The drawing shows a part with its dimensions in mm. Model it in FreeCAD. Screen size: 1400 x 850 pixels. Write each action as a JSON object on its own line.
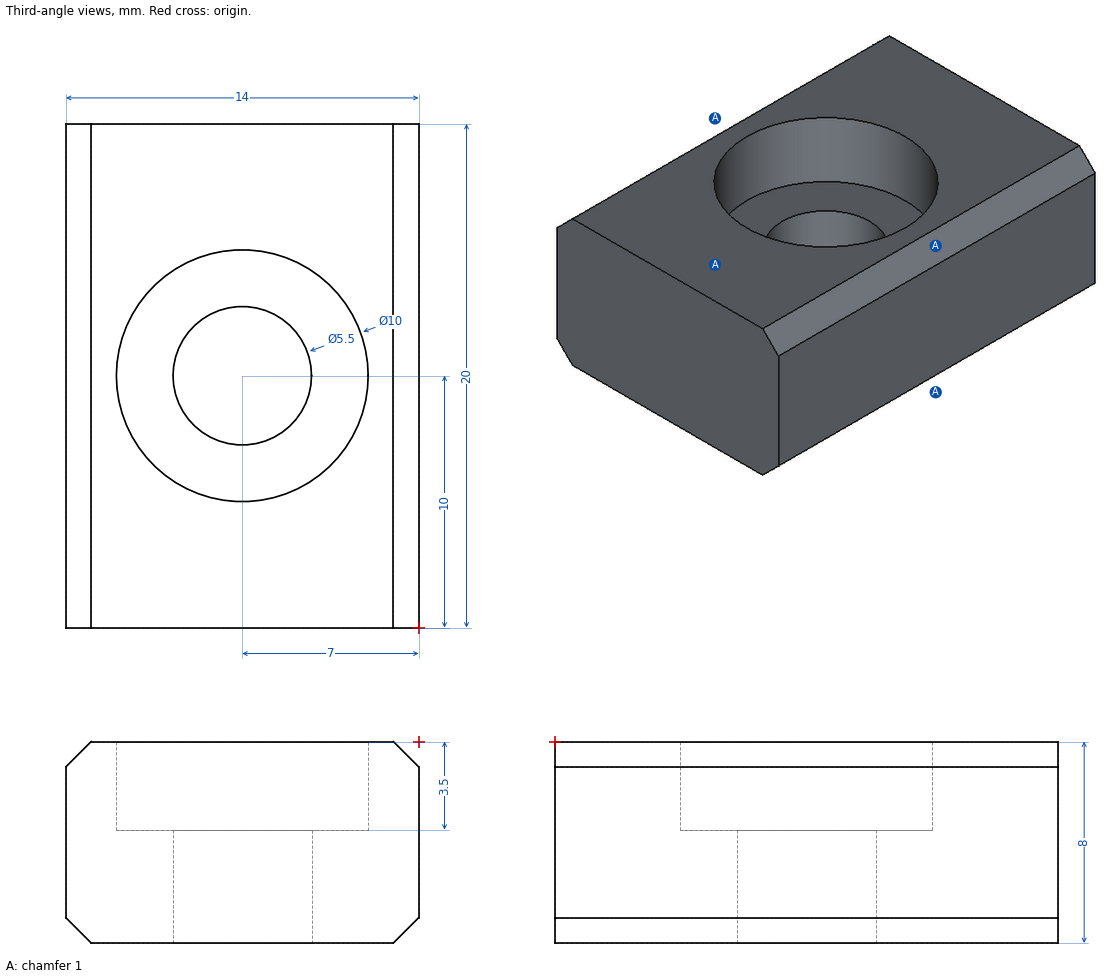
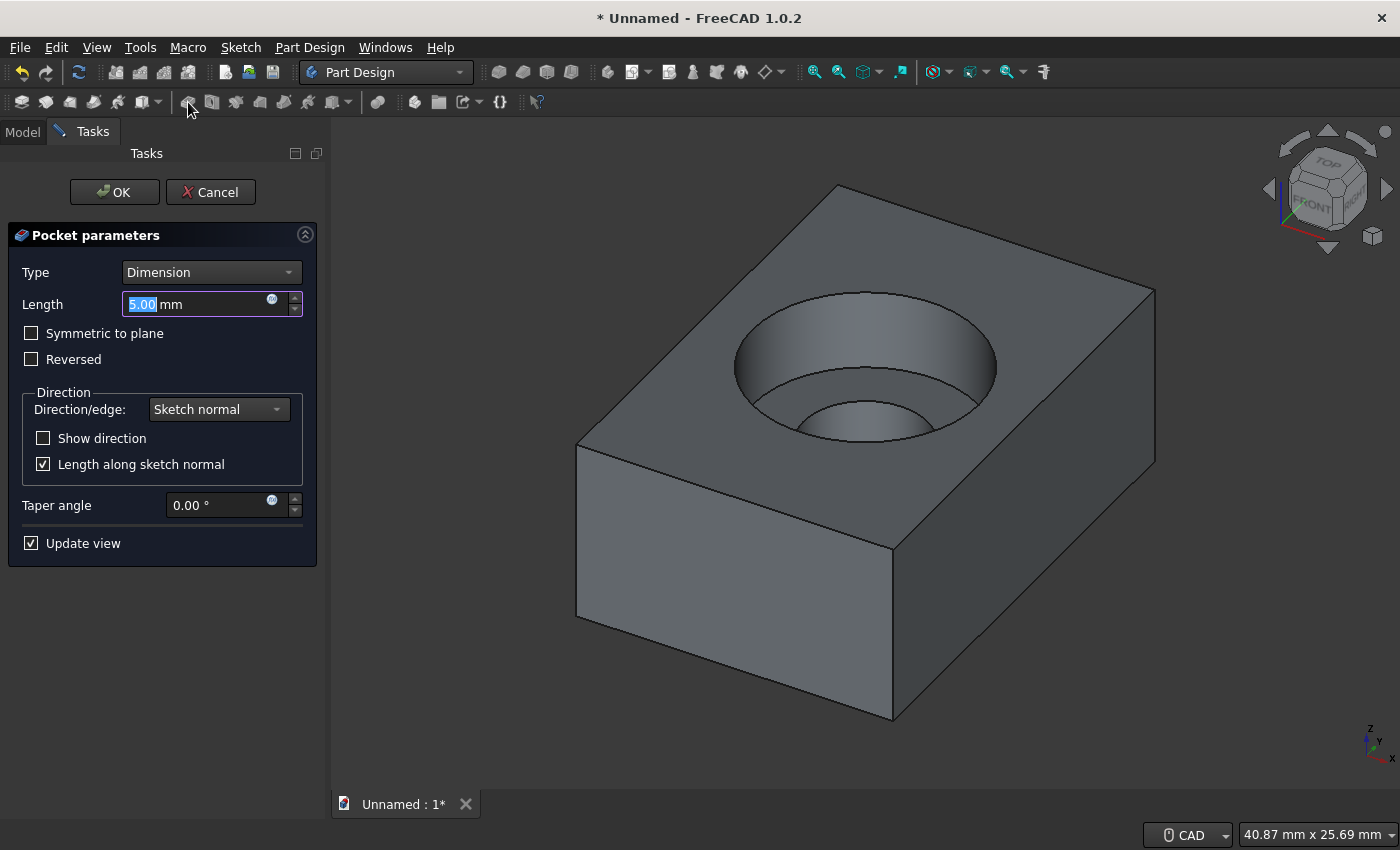
{"action": "left_click", "coordinate": [212, 272]}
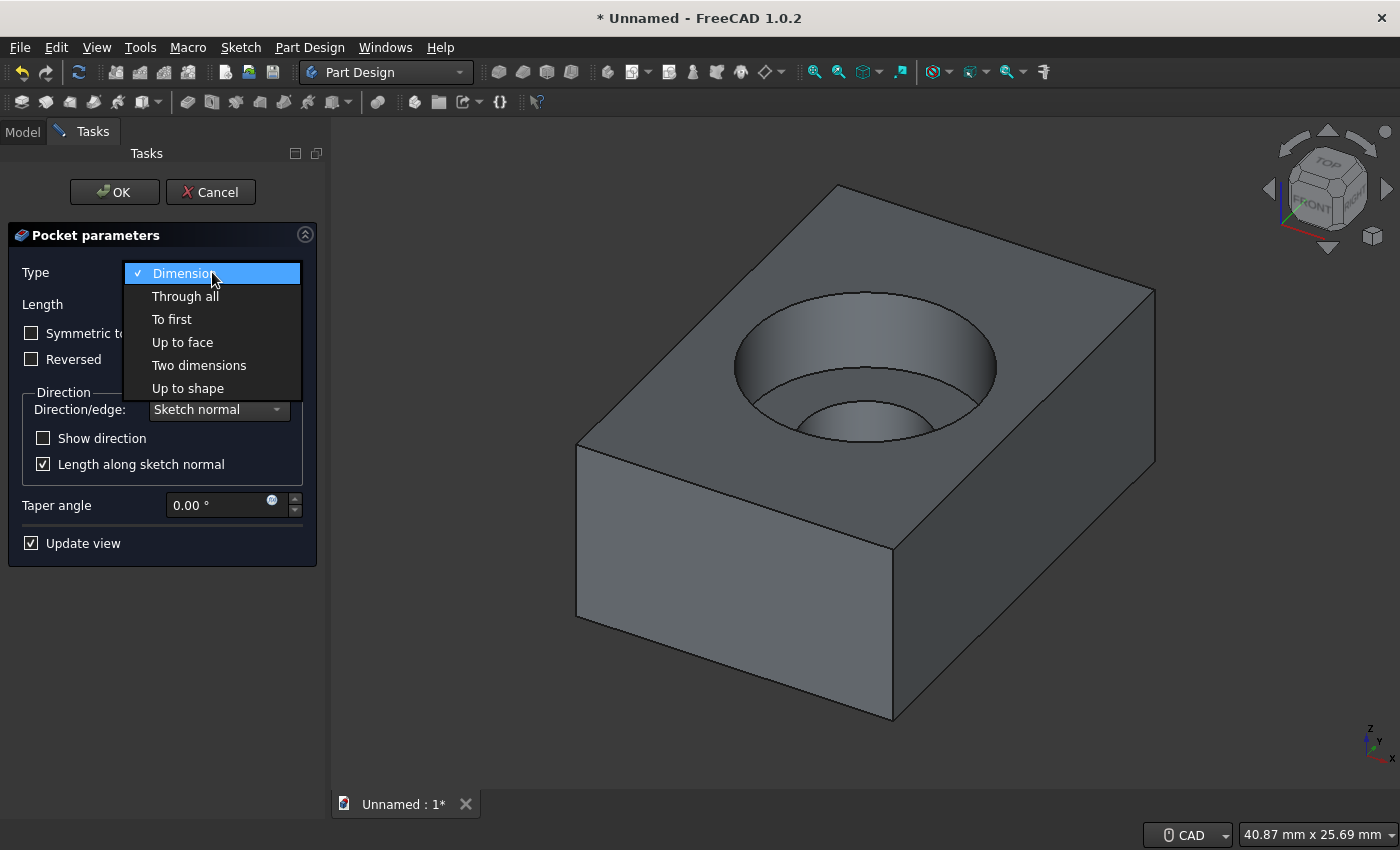
{"action": "left_click", "coordinate": [212, 296]}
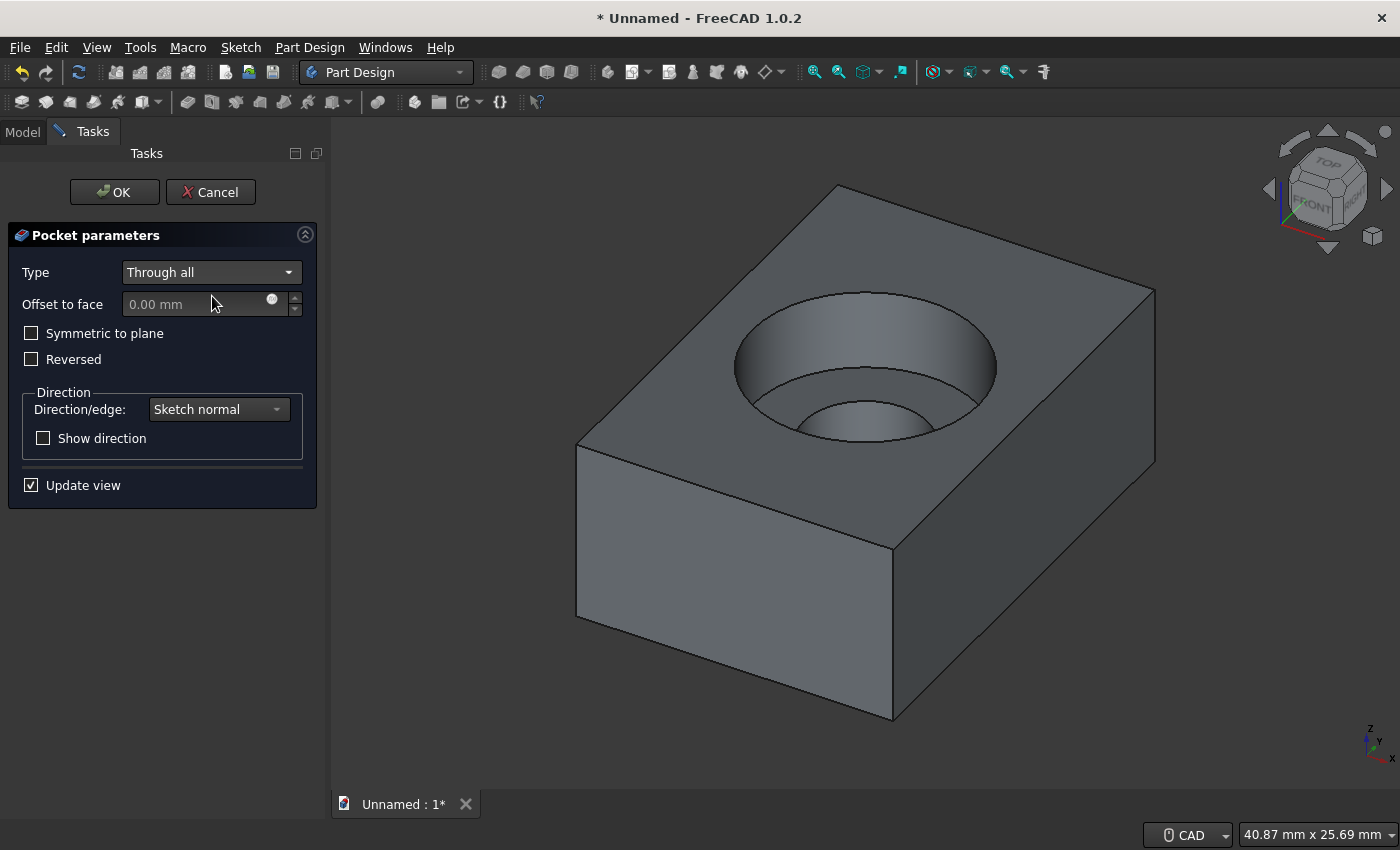
{"action": "left_click", "coordinate": [115, 192]}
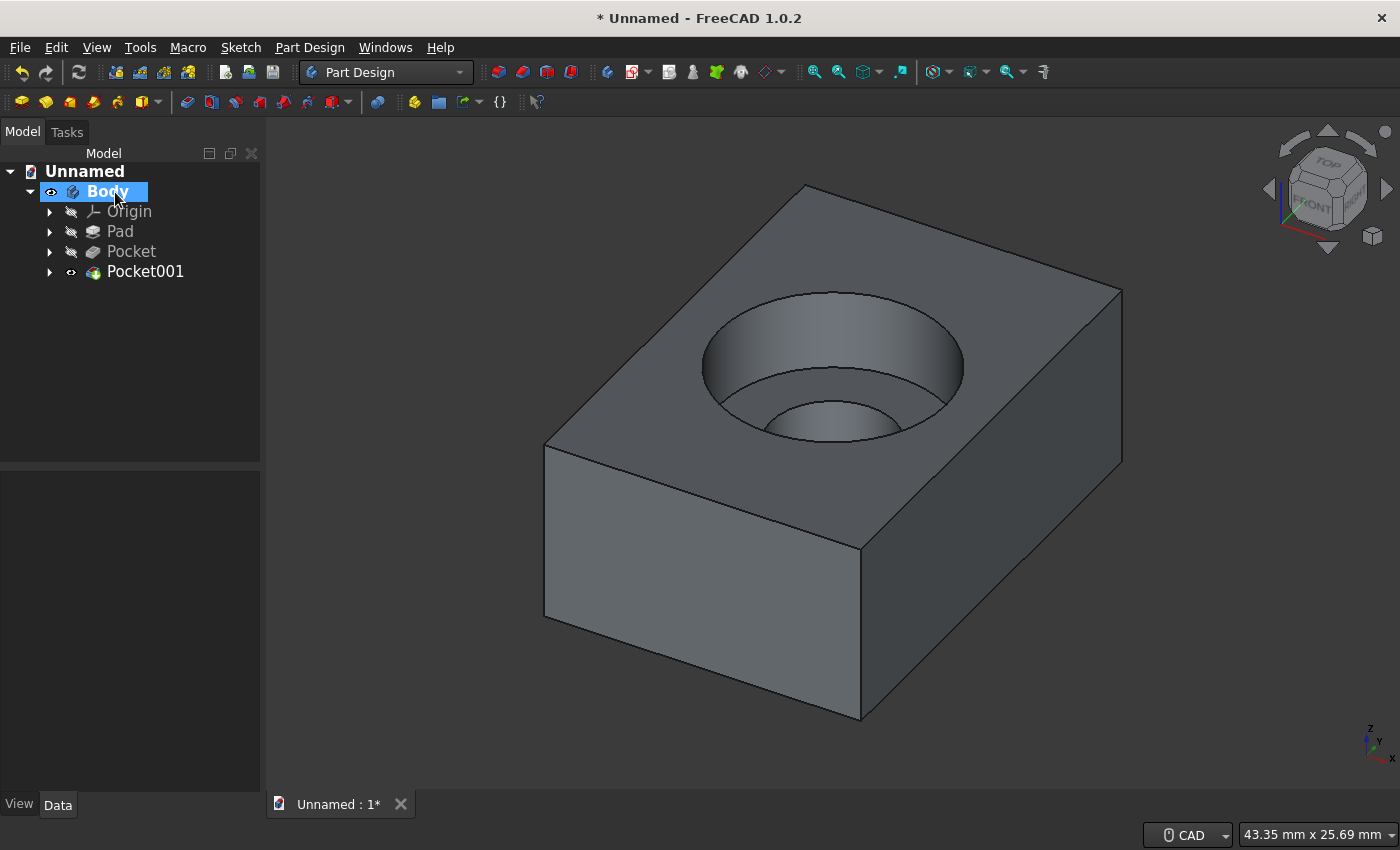
{"action": "left_click", "coordinate": [992, 419]}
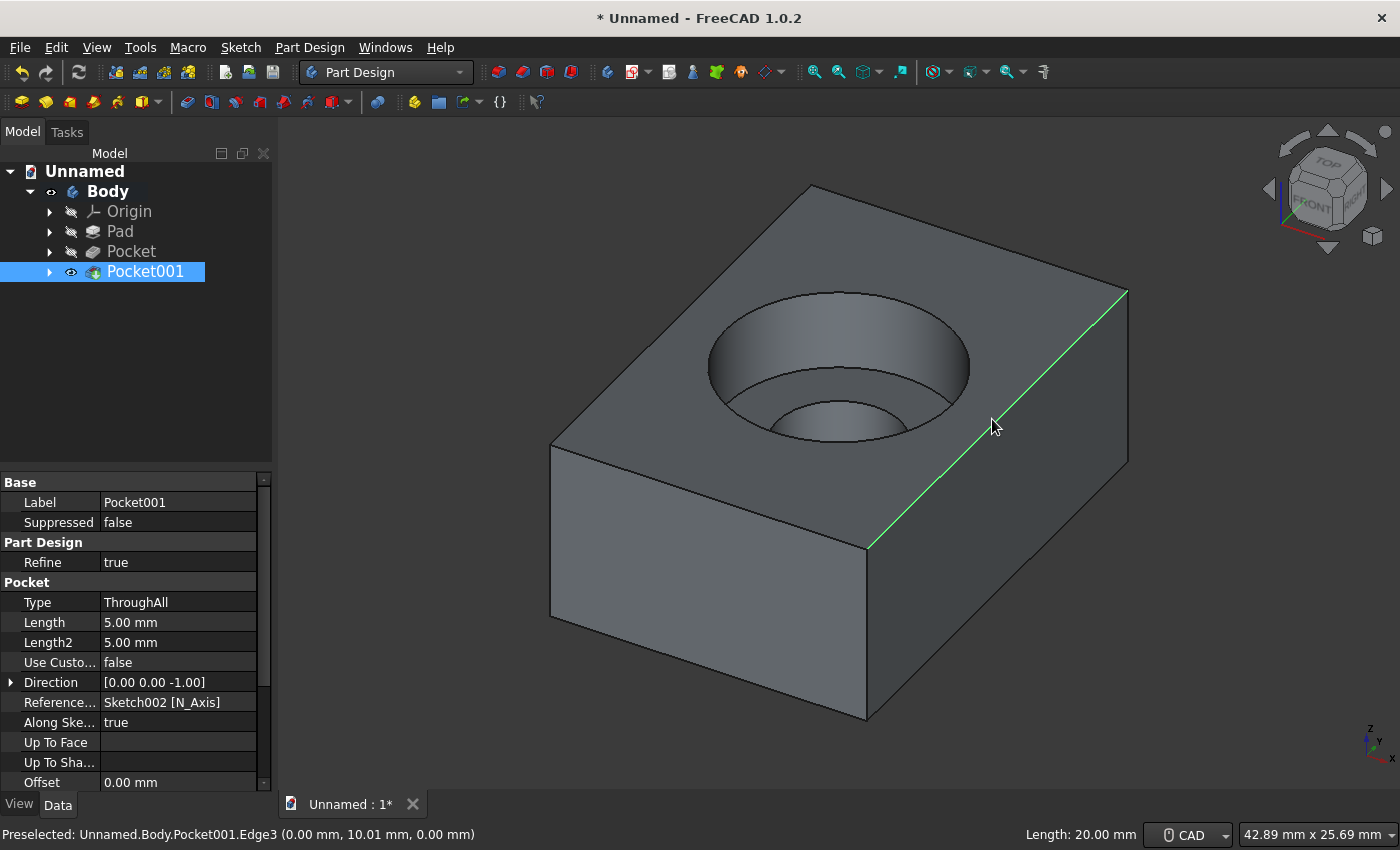
{"action": "key", "text": "0"}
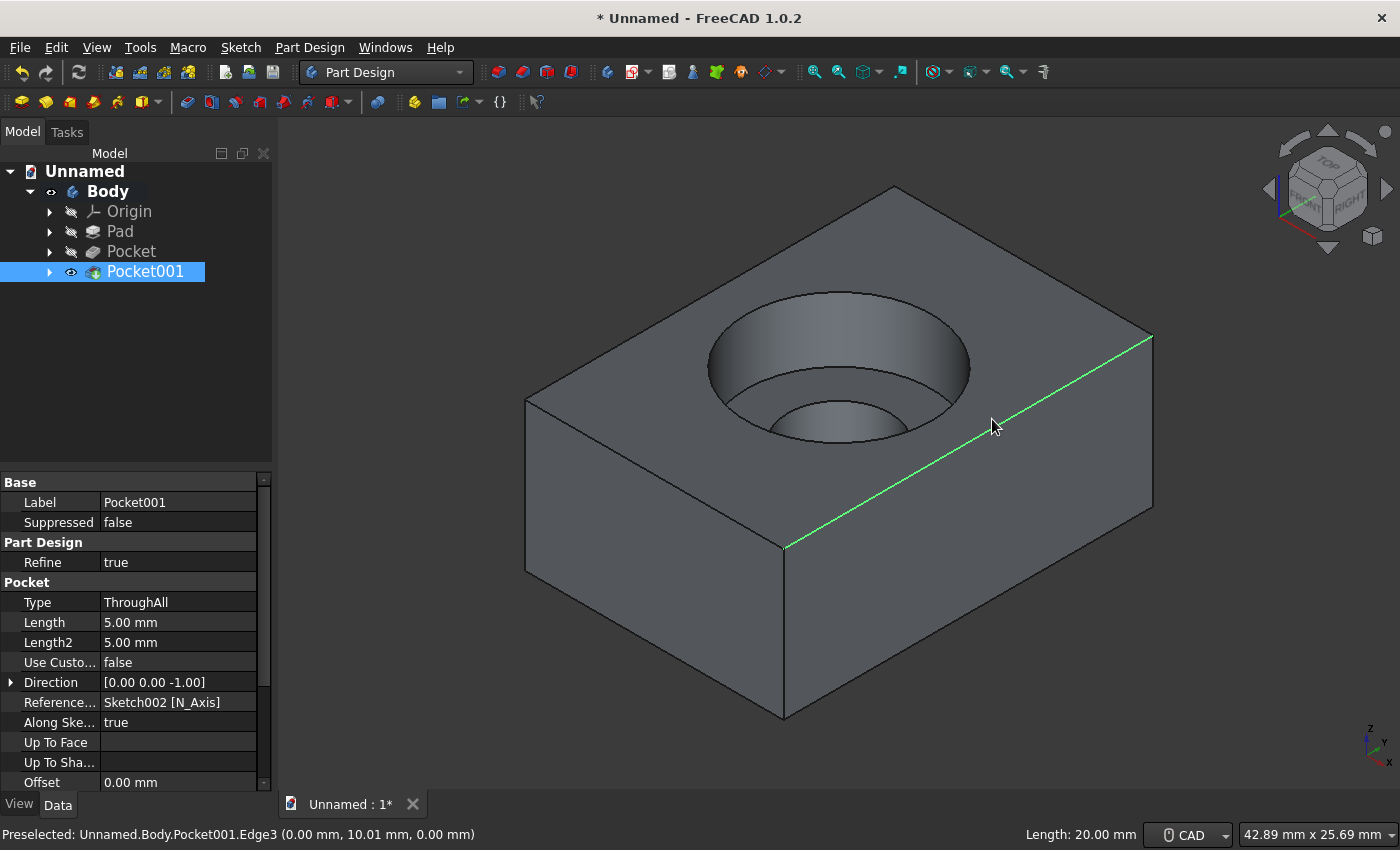
{"action": "key", "text": "2"}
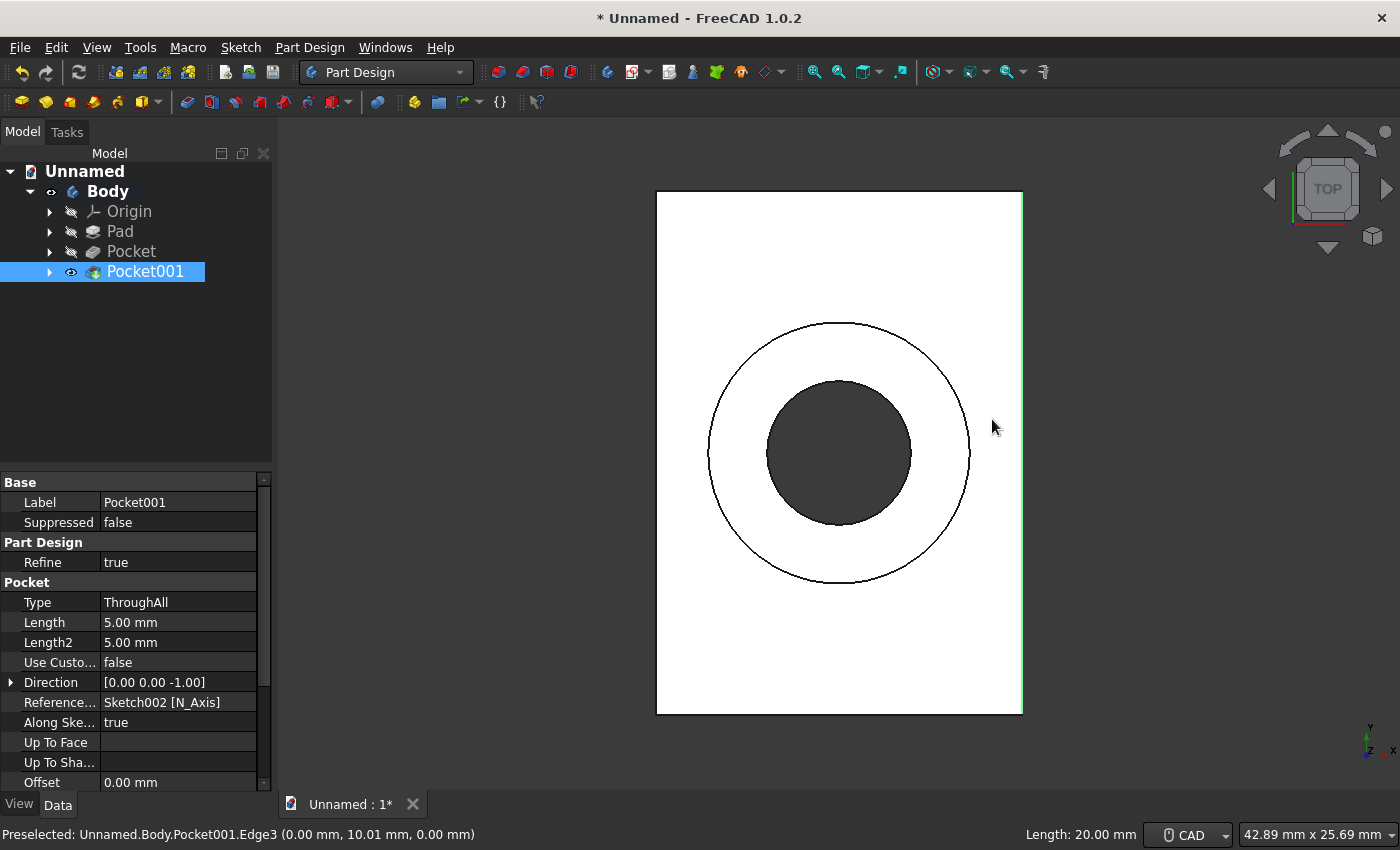
{"action": "left_click", "coordinate": [656, 452], "text": "ctrl"}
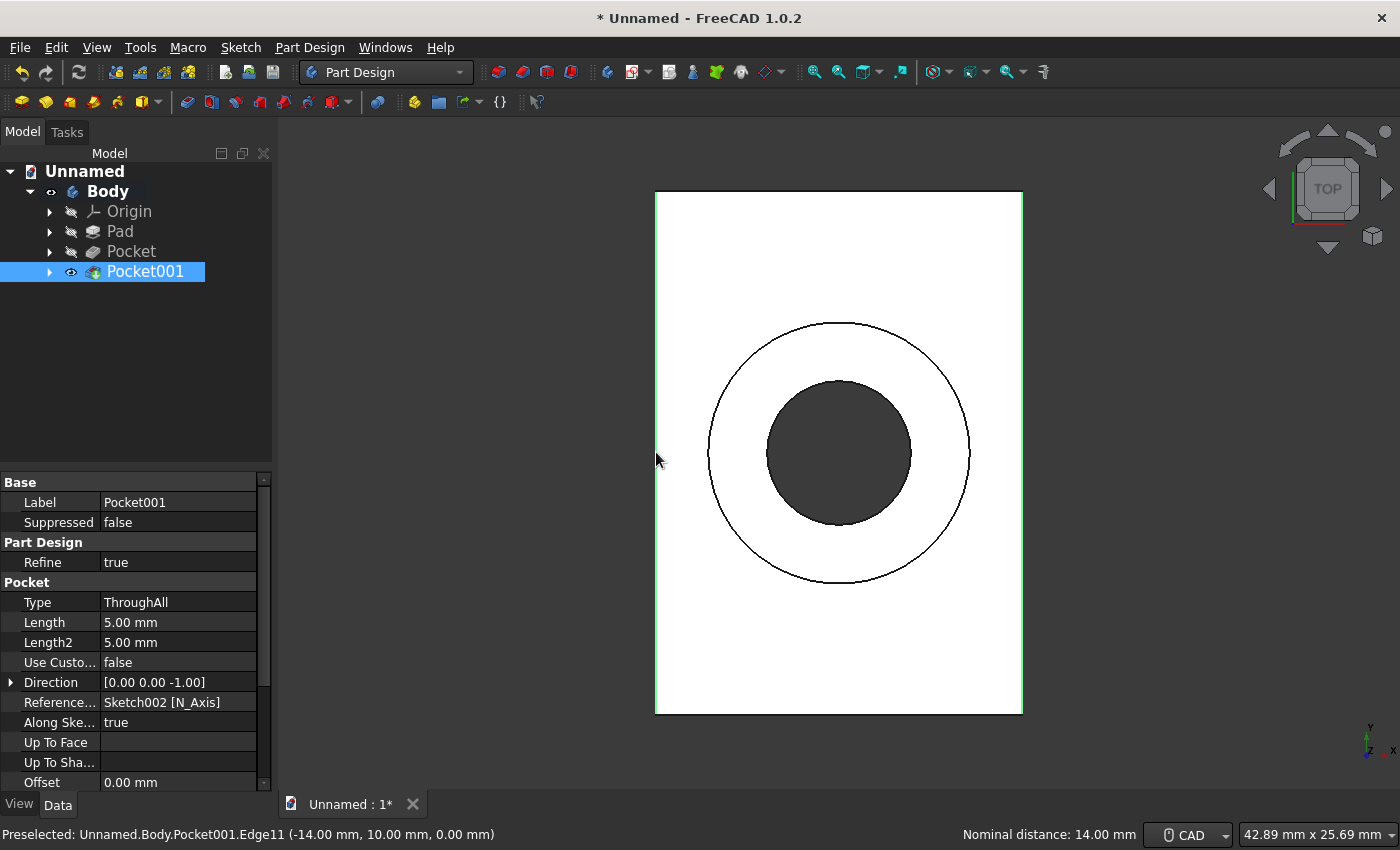
{"action": "key", "text": "1"}